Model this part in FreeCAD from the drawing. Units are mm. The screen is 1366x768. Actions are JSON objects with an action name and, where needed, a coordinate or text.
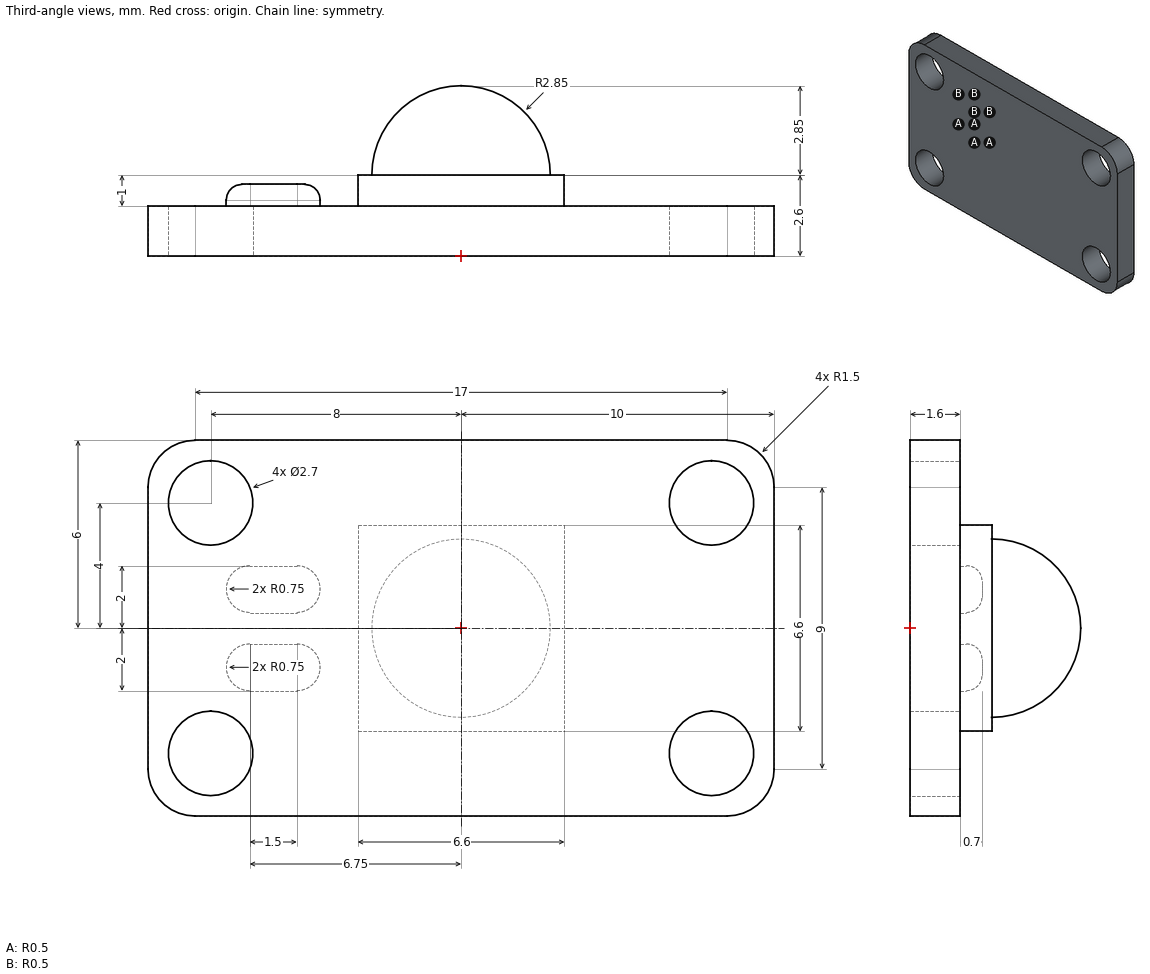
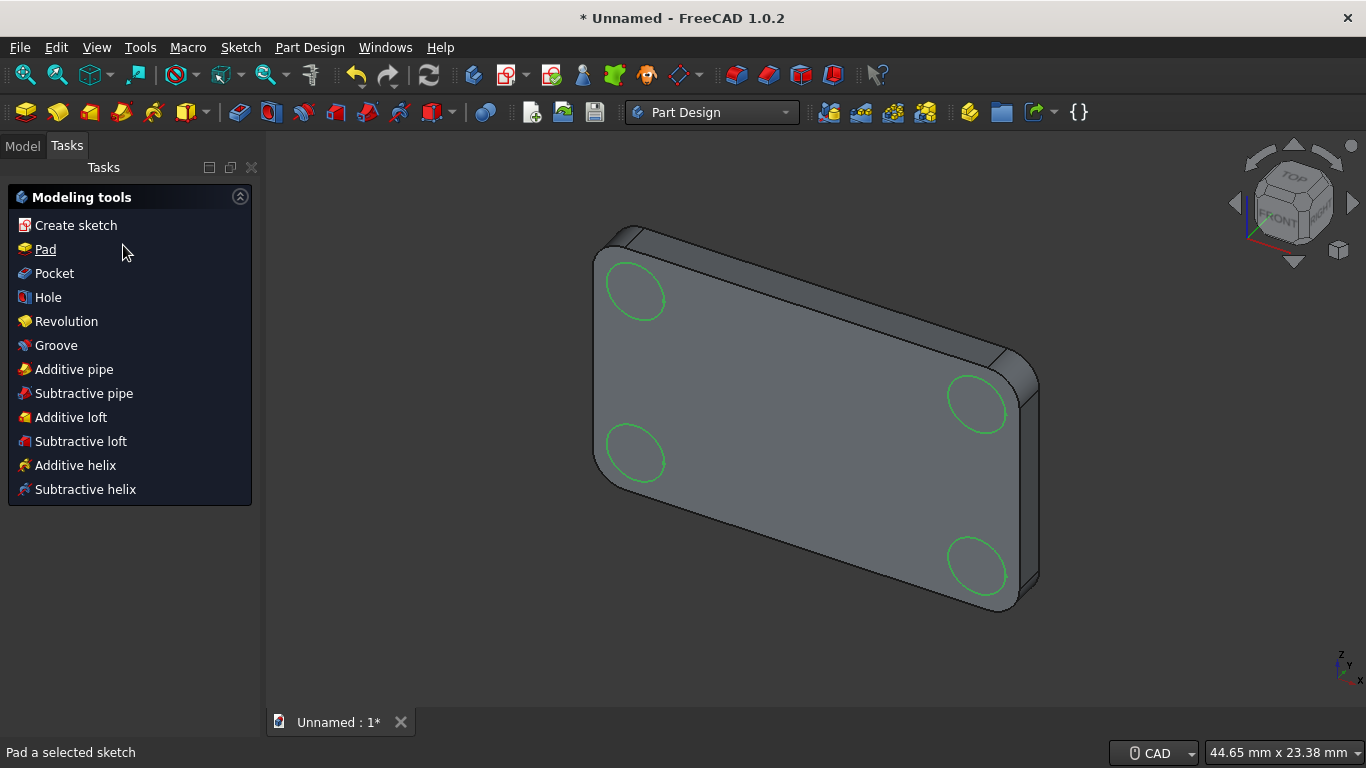
{"action": "left_click", "coordinate": [240, 112]}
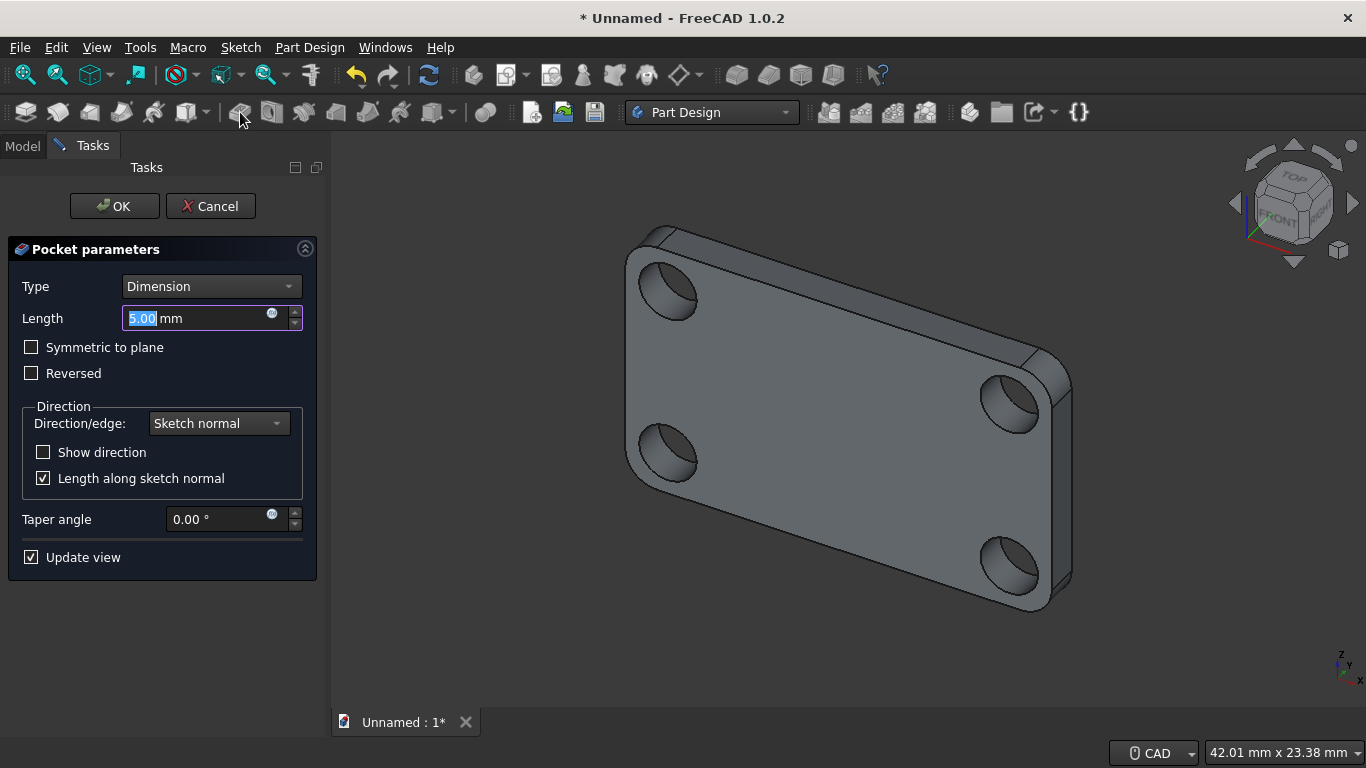
{"action": "left_click", "coordinate": [212, 286]}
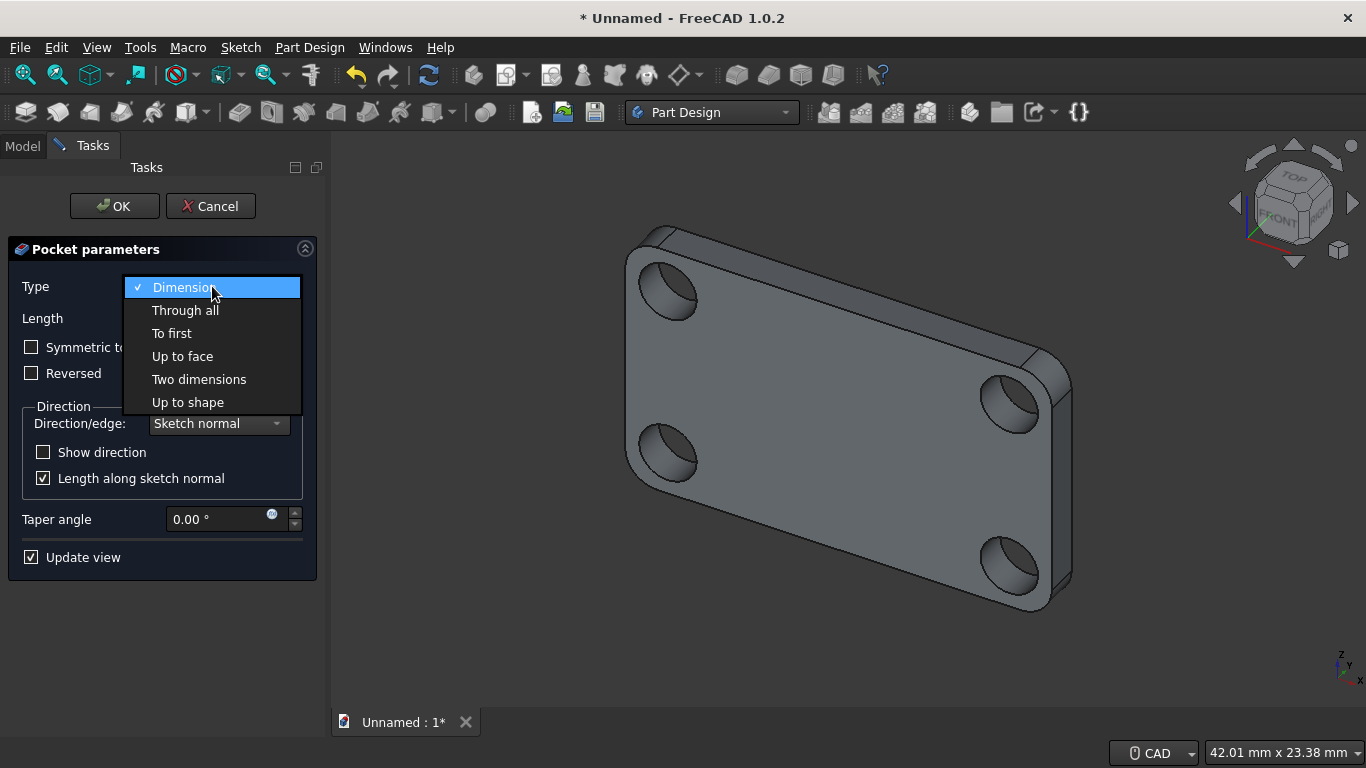
{"action": "left_click", "coordinate": [212, 310]}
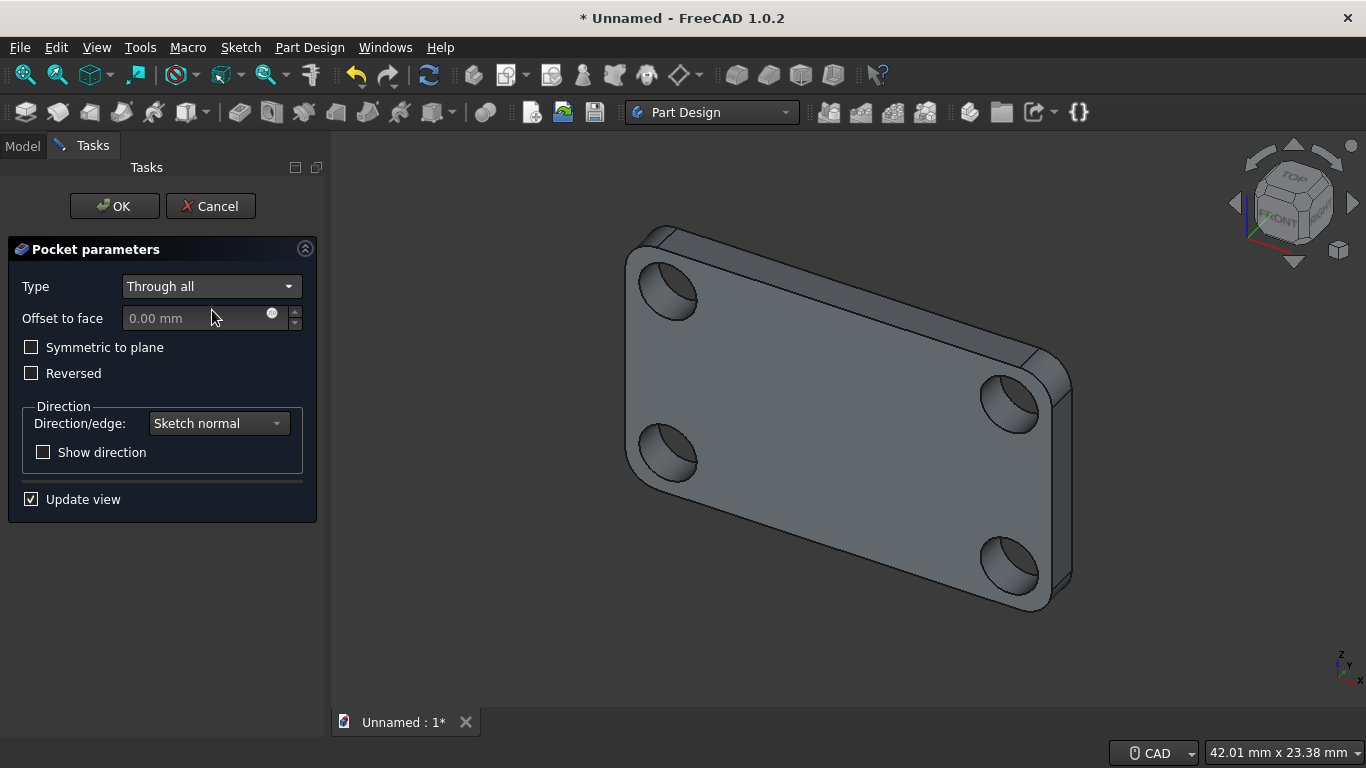
{"action": "left_click", "coordinate": [115, 206]}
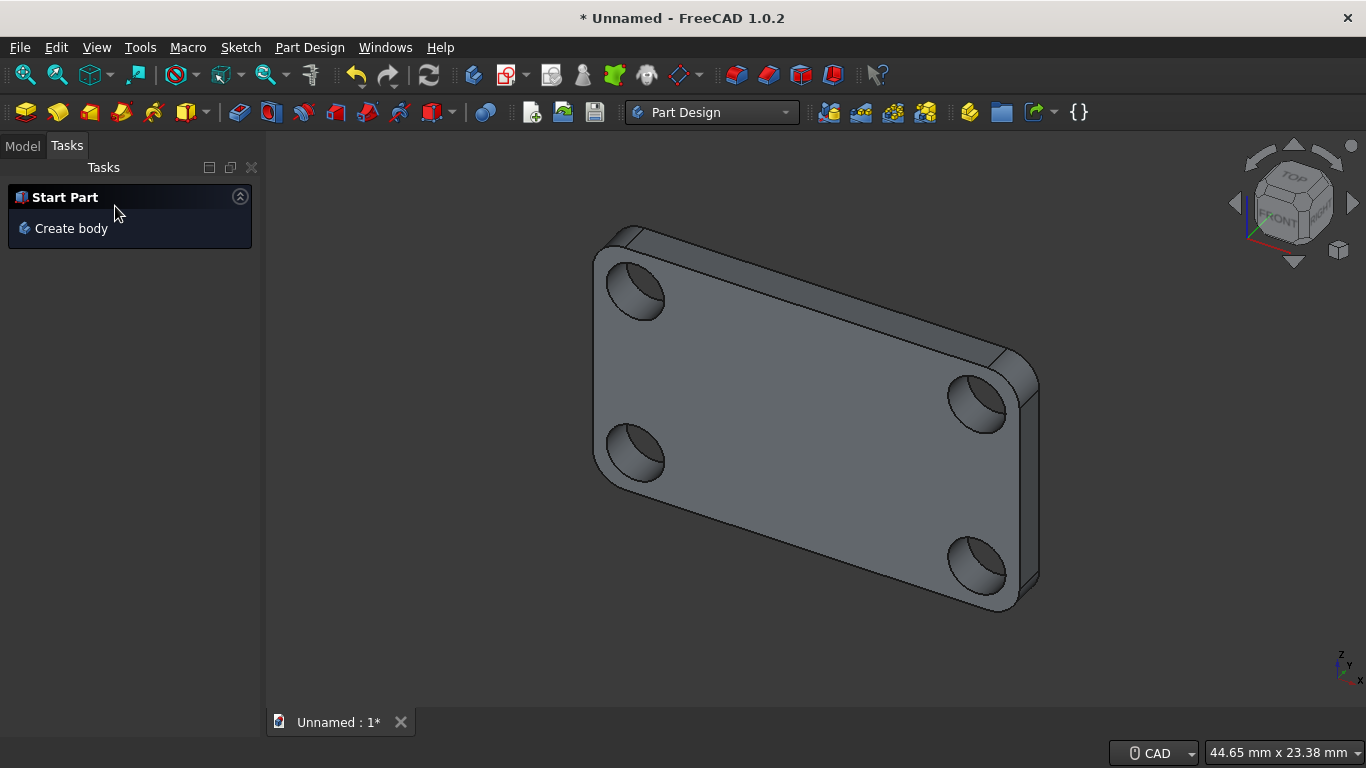
{"action": "left_click", "coordinate": [474, 76]}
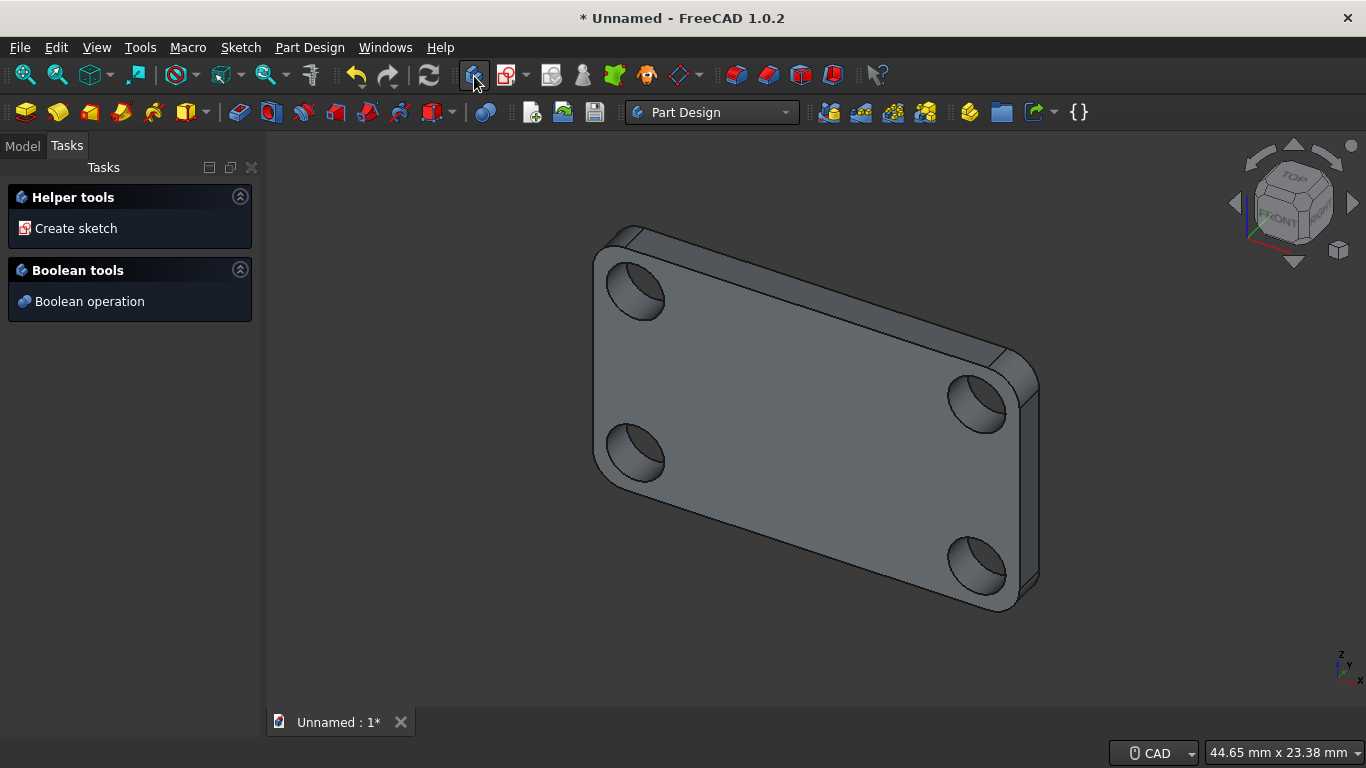
{"action": "left_click", "coordinate": [23, 145]}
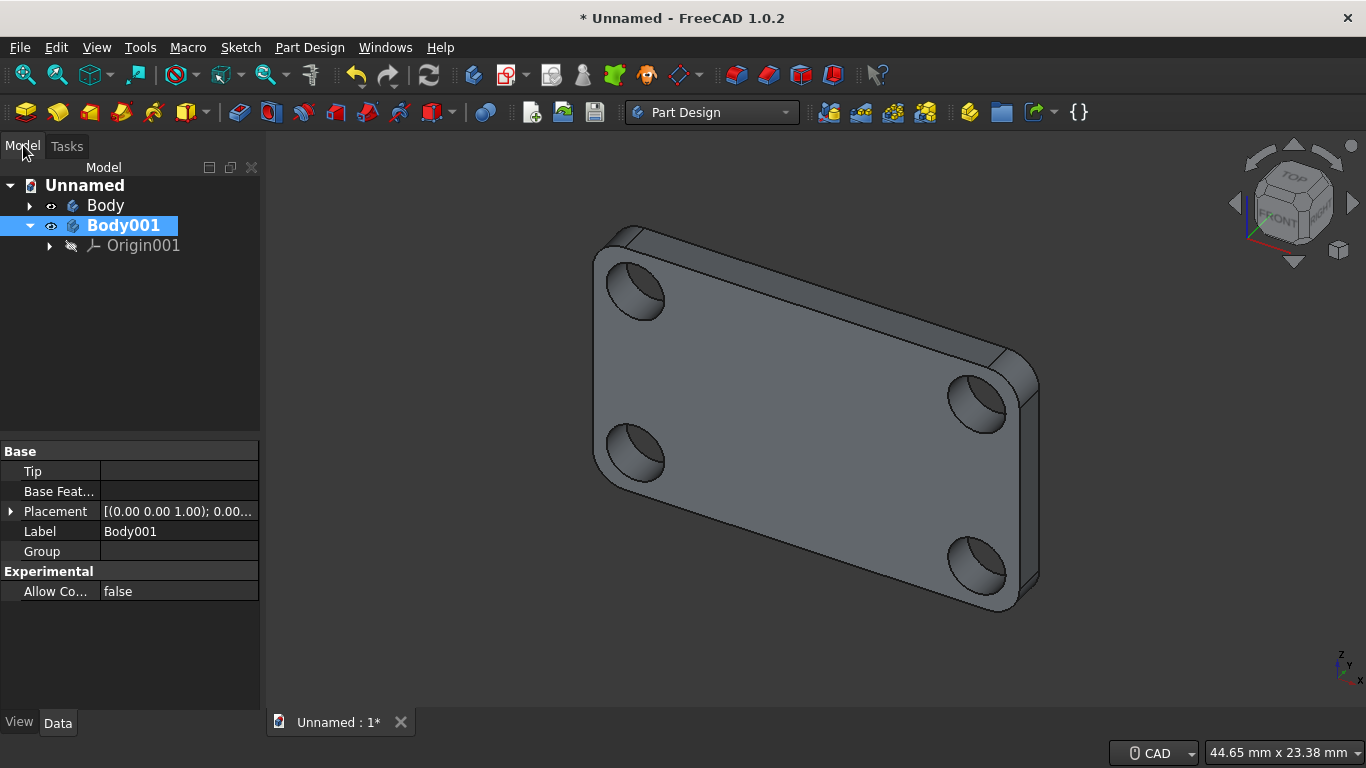
{"action": "left_click", "coordinate": [50, 246]}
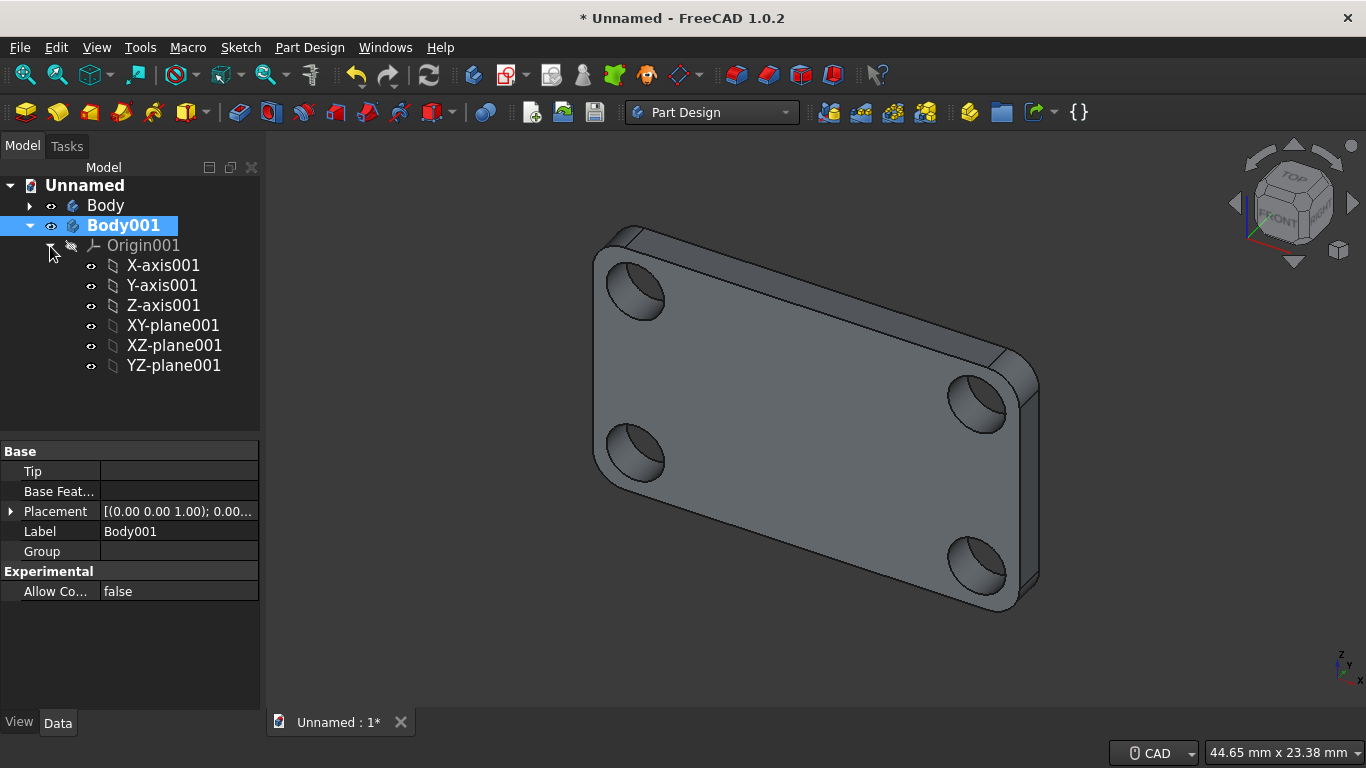
{"action": "left_click", "coordinate": [136, 346]}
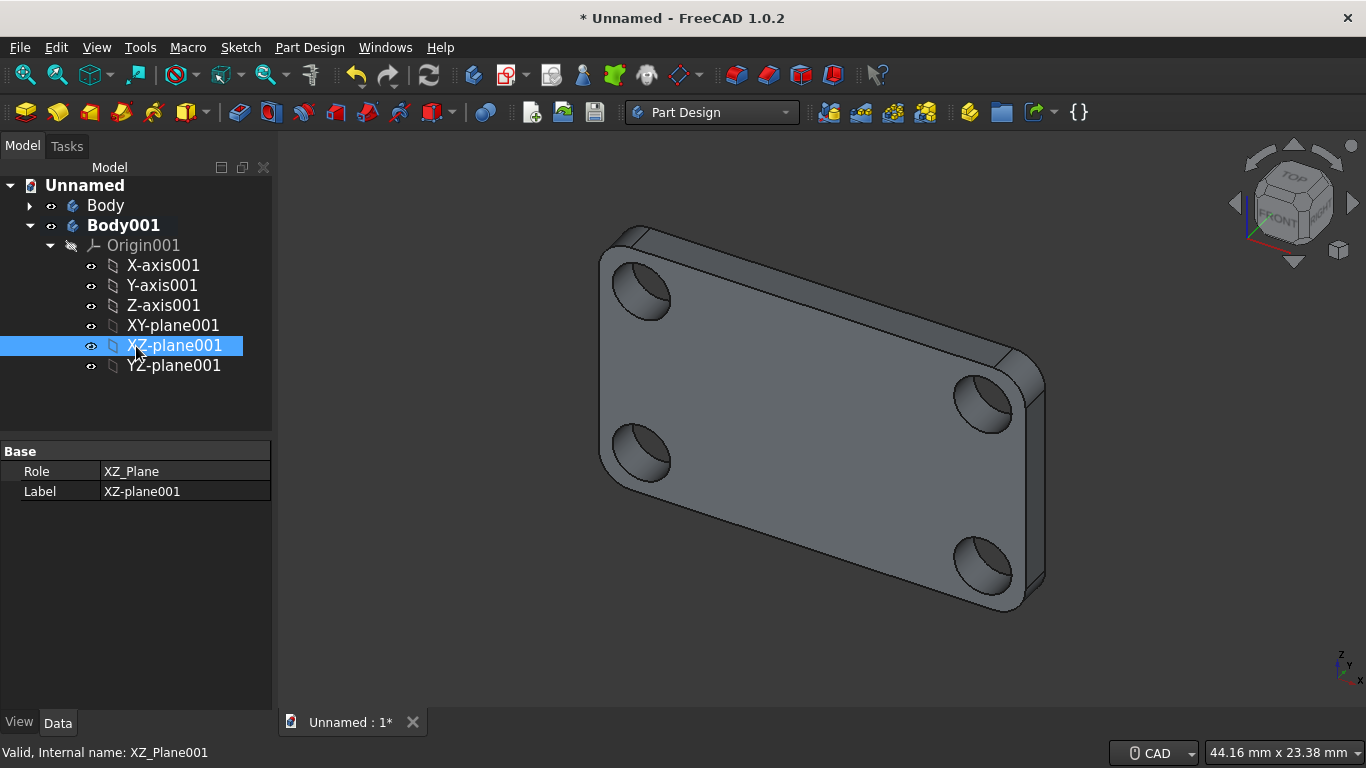
{"action": "left_click", "coordinate": [680, 76]}